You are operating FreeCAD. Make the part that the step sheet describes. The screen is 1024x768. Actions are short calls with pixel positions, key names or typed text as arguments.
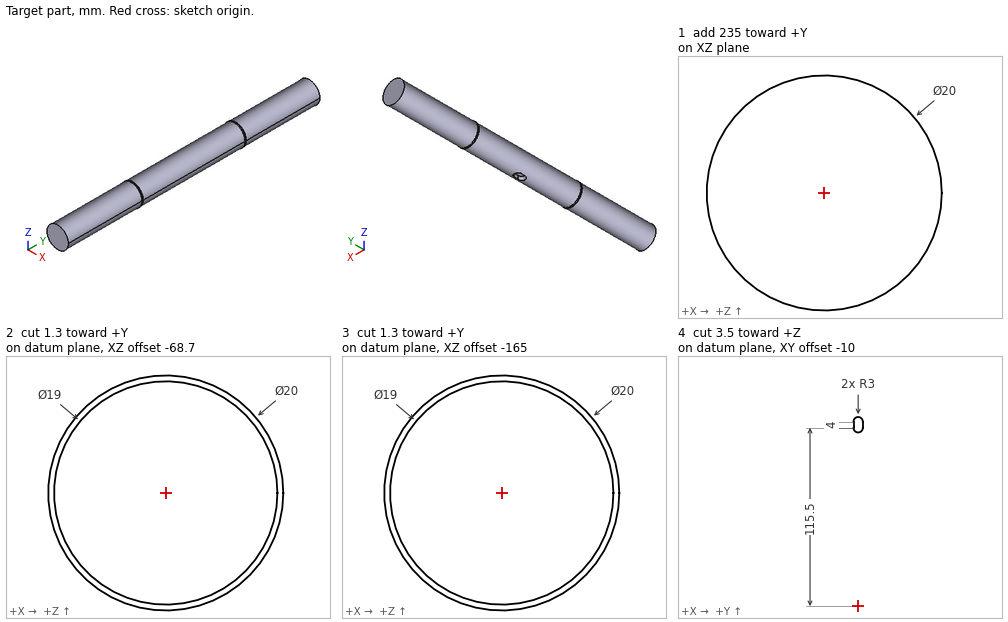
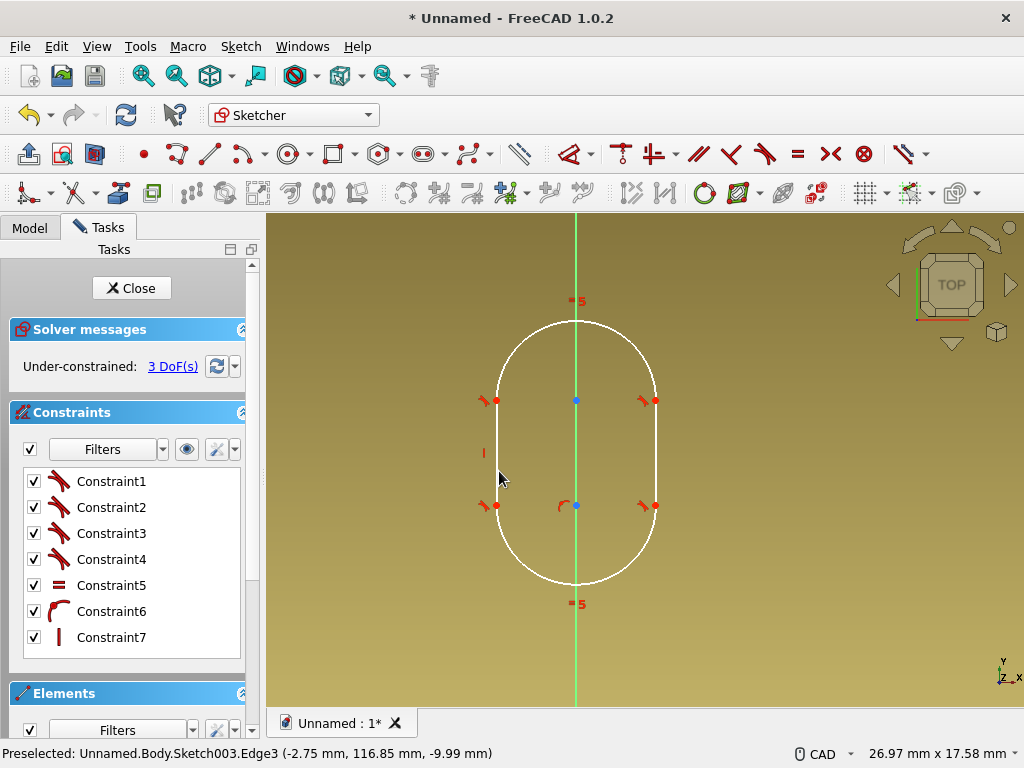
click(530, 569)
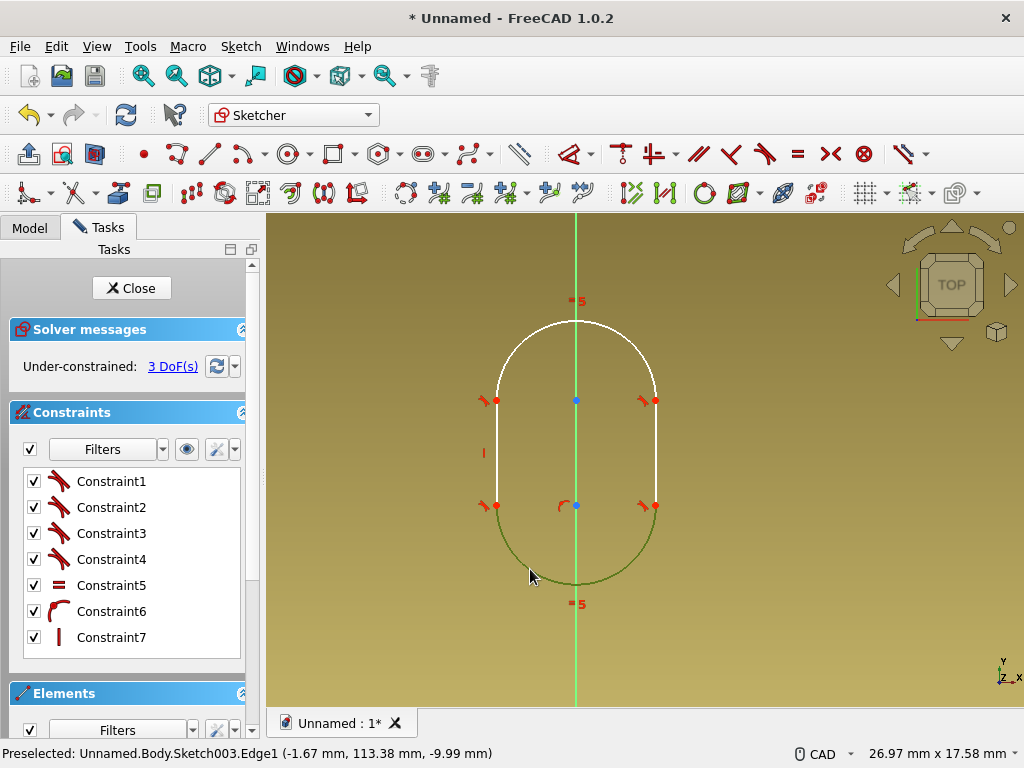
key(k)
key(r)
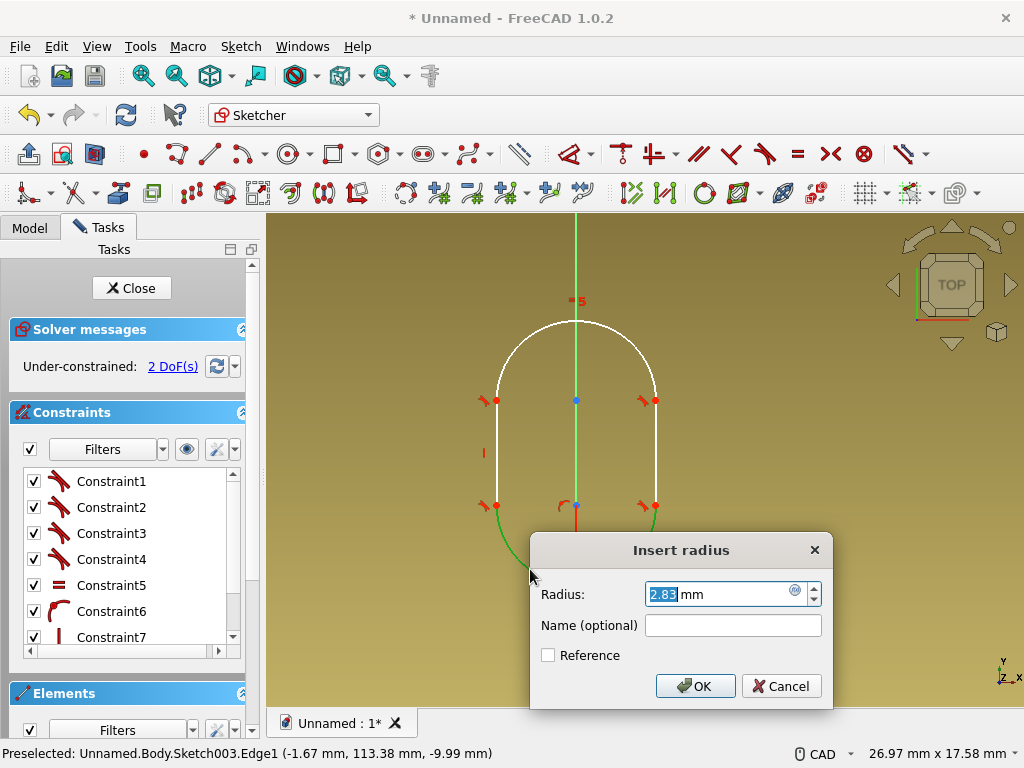
text(3)
key(Return)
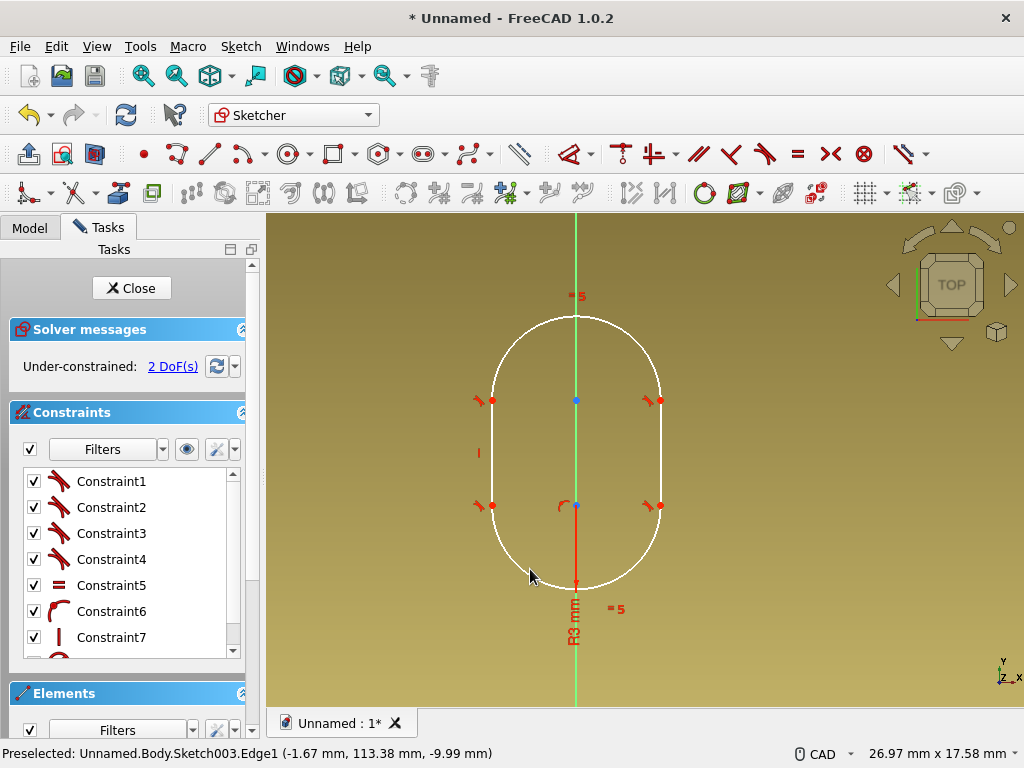
click(492, 474)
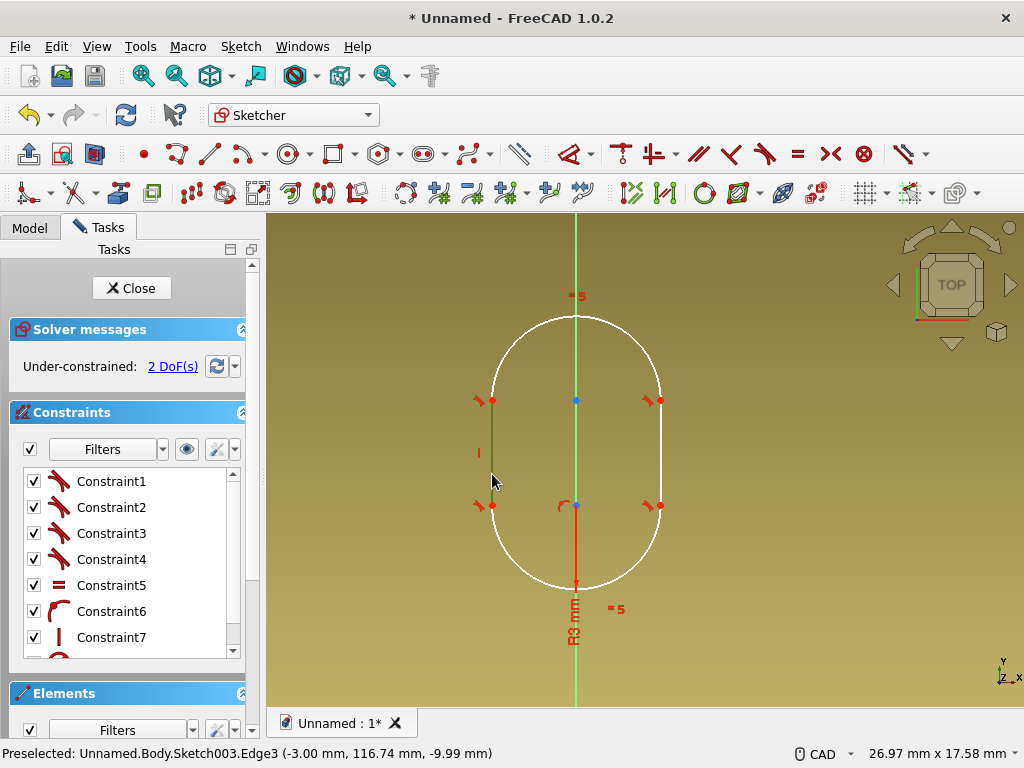
key(i)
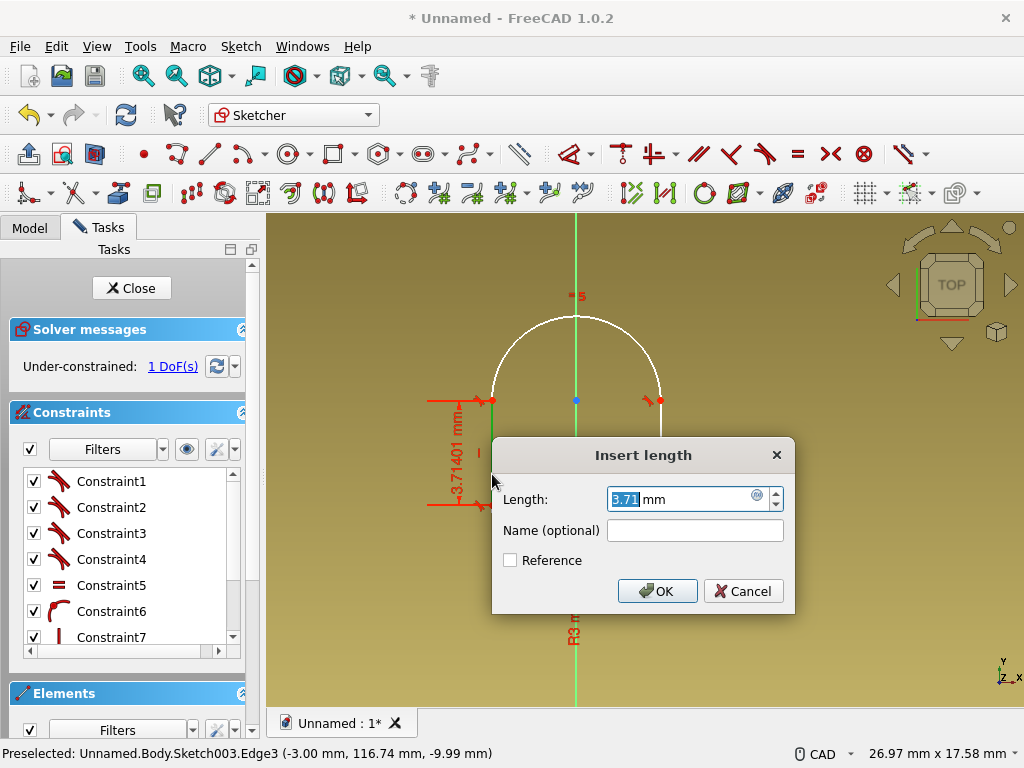
text(4)
key(Return)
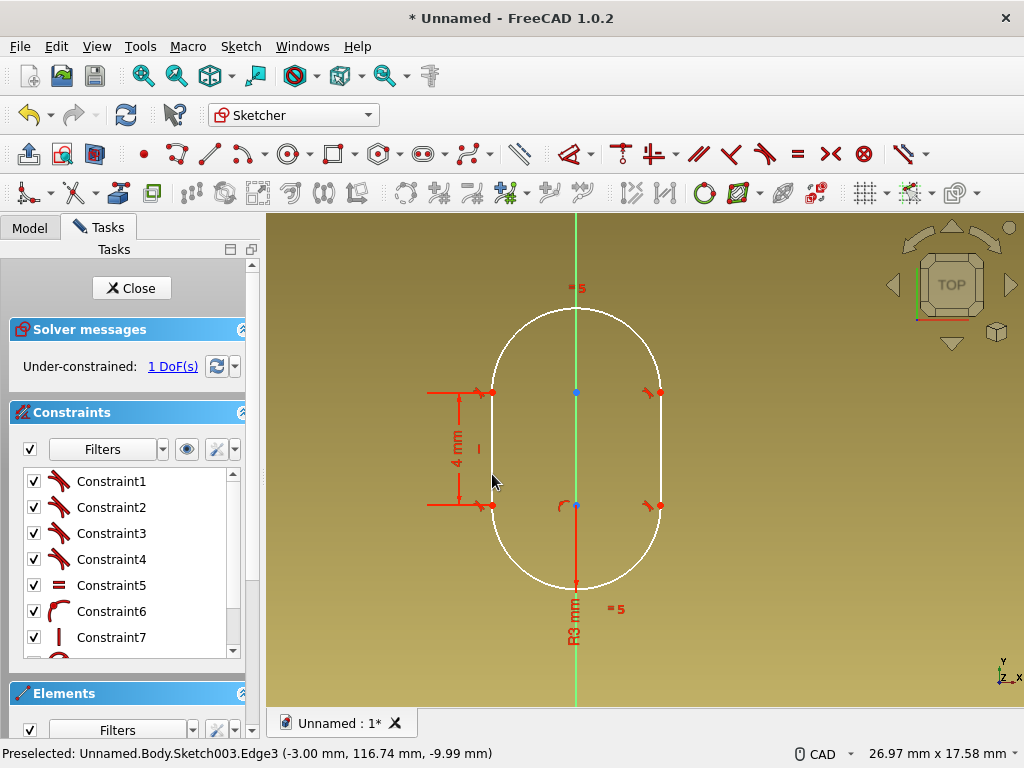
click(492, 505)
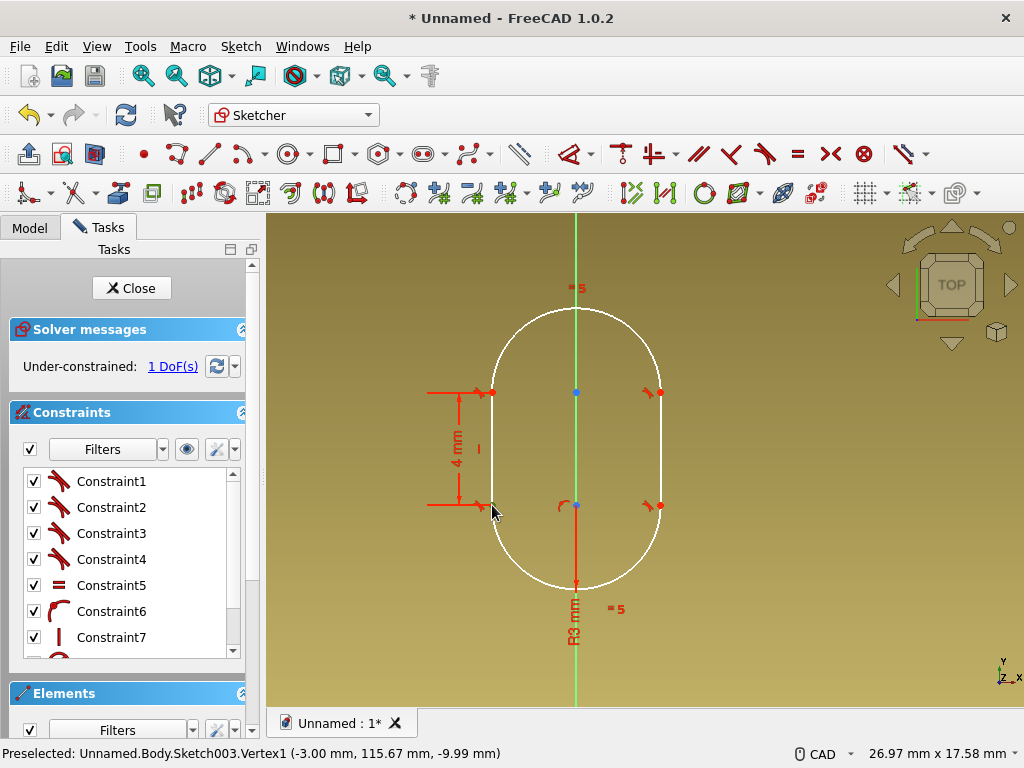
click(590, 154)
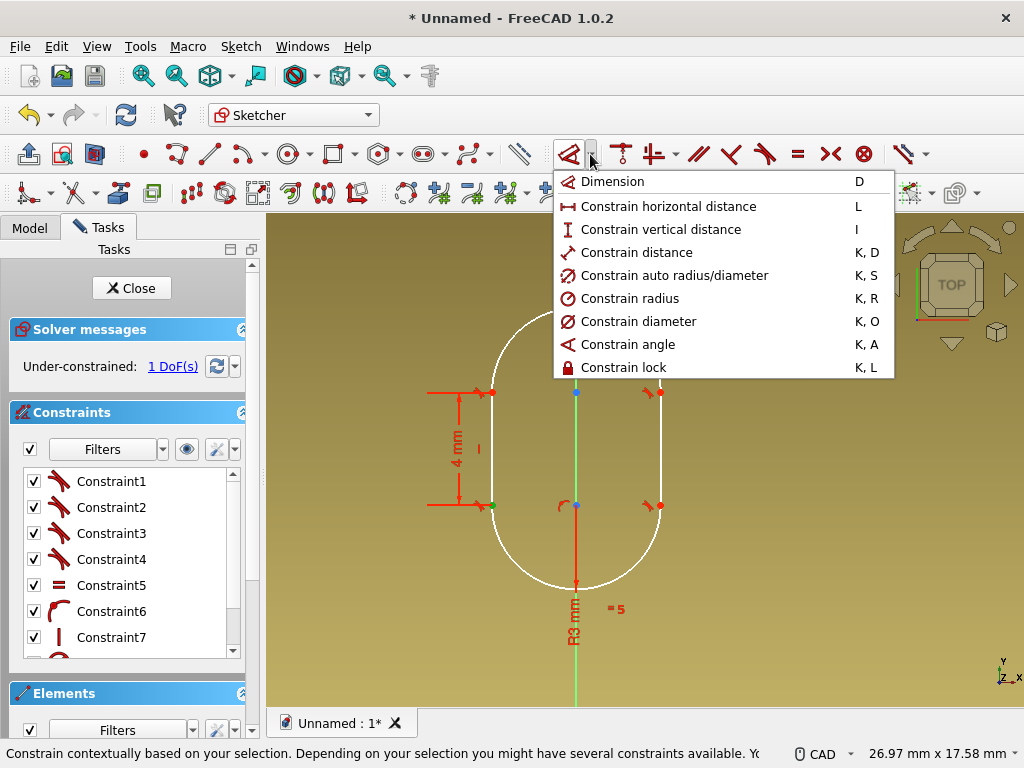
click(724, 230)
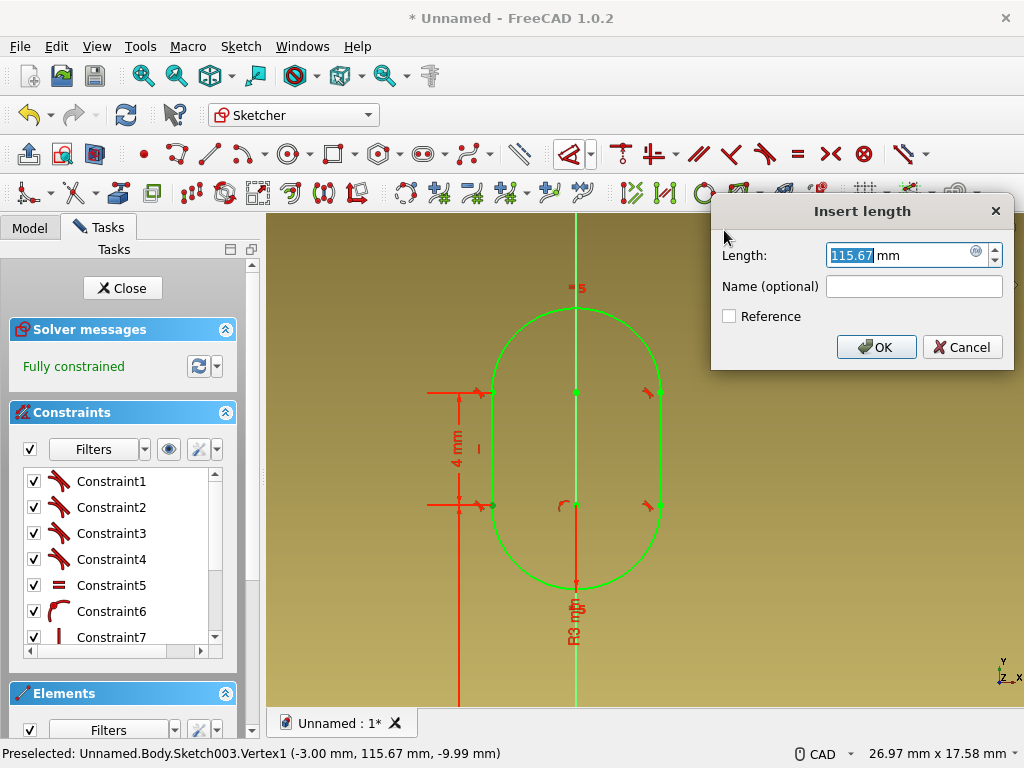
text(115.5)
key(Return)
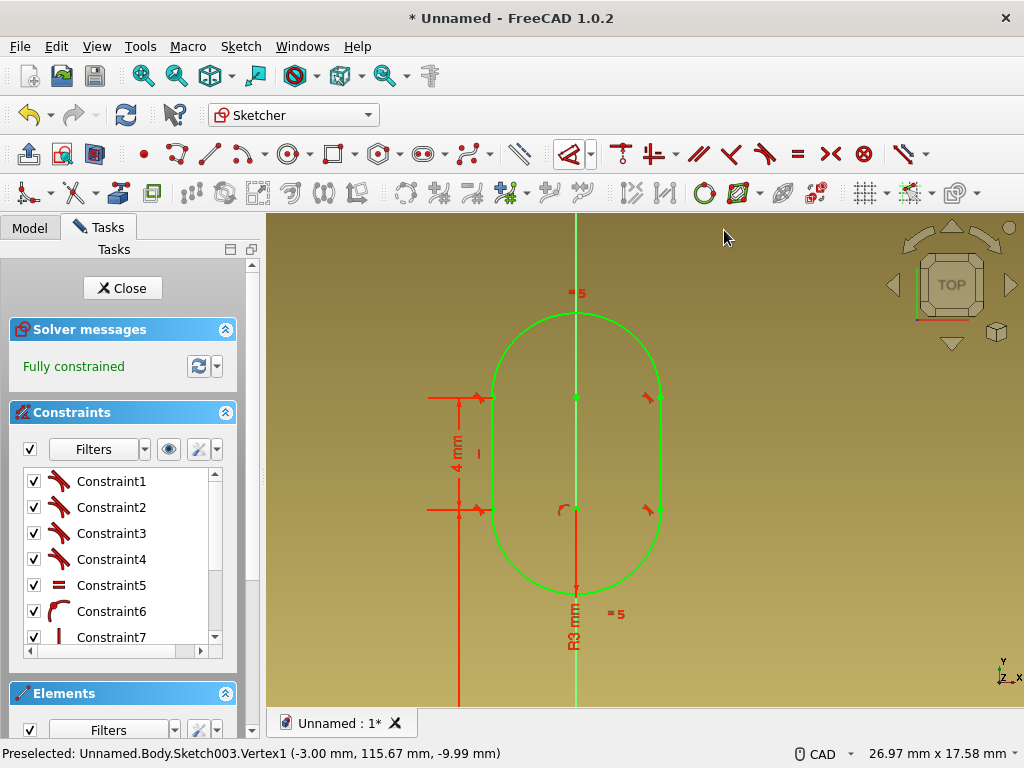
click(123, 288)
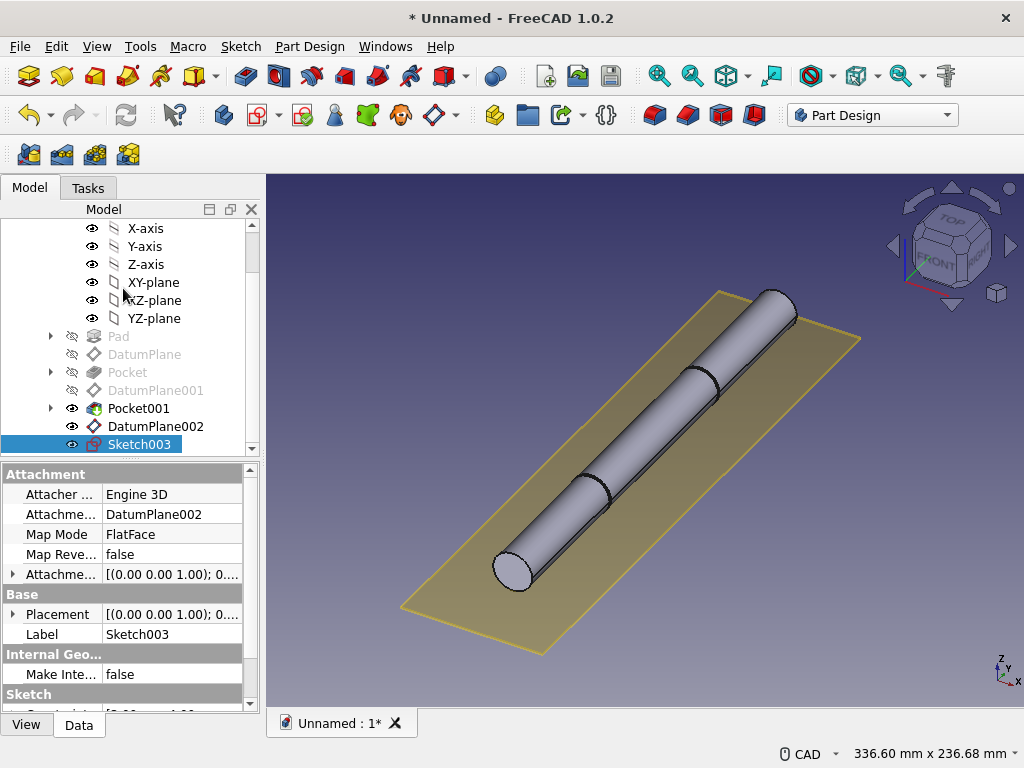
click(246, 76)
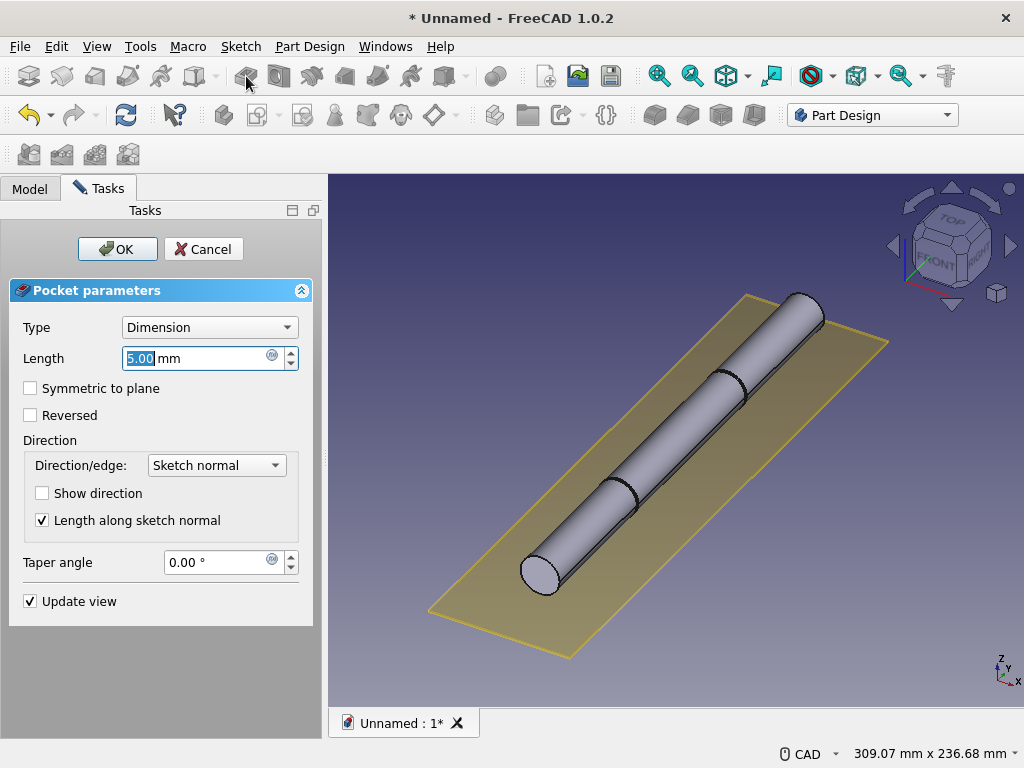
text(3.5)
key(Tab)